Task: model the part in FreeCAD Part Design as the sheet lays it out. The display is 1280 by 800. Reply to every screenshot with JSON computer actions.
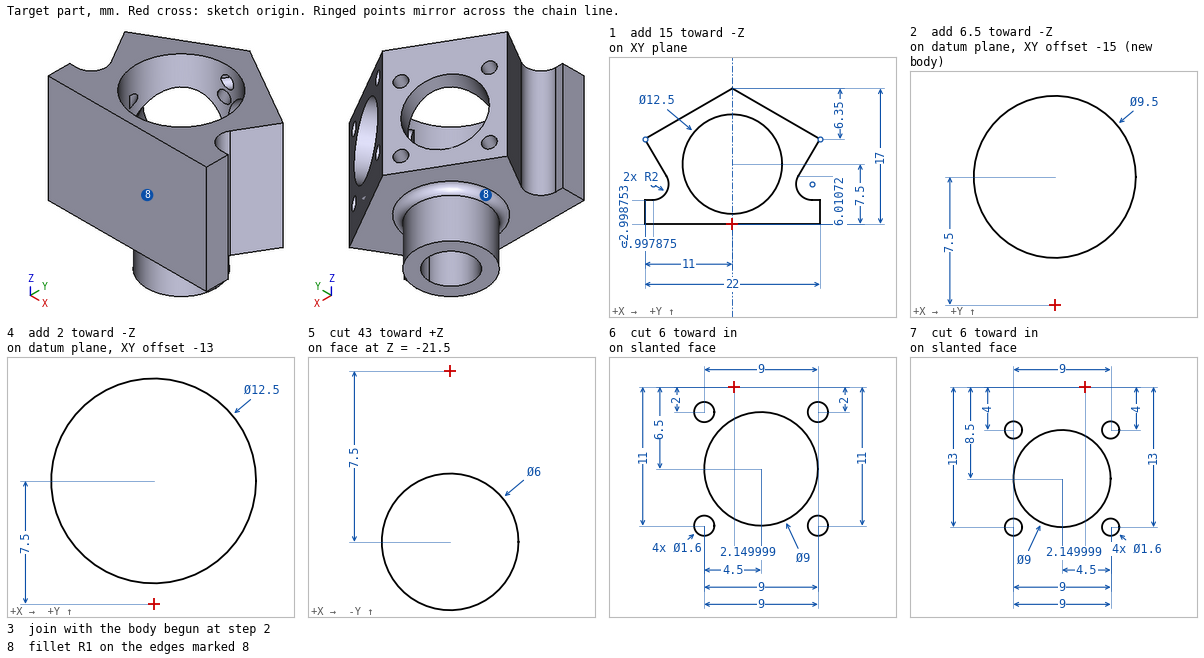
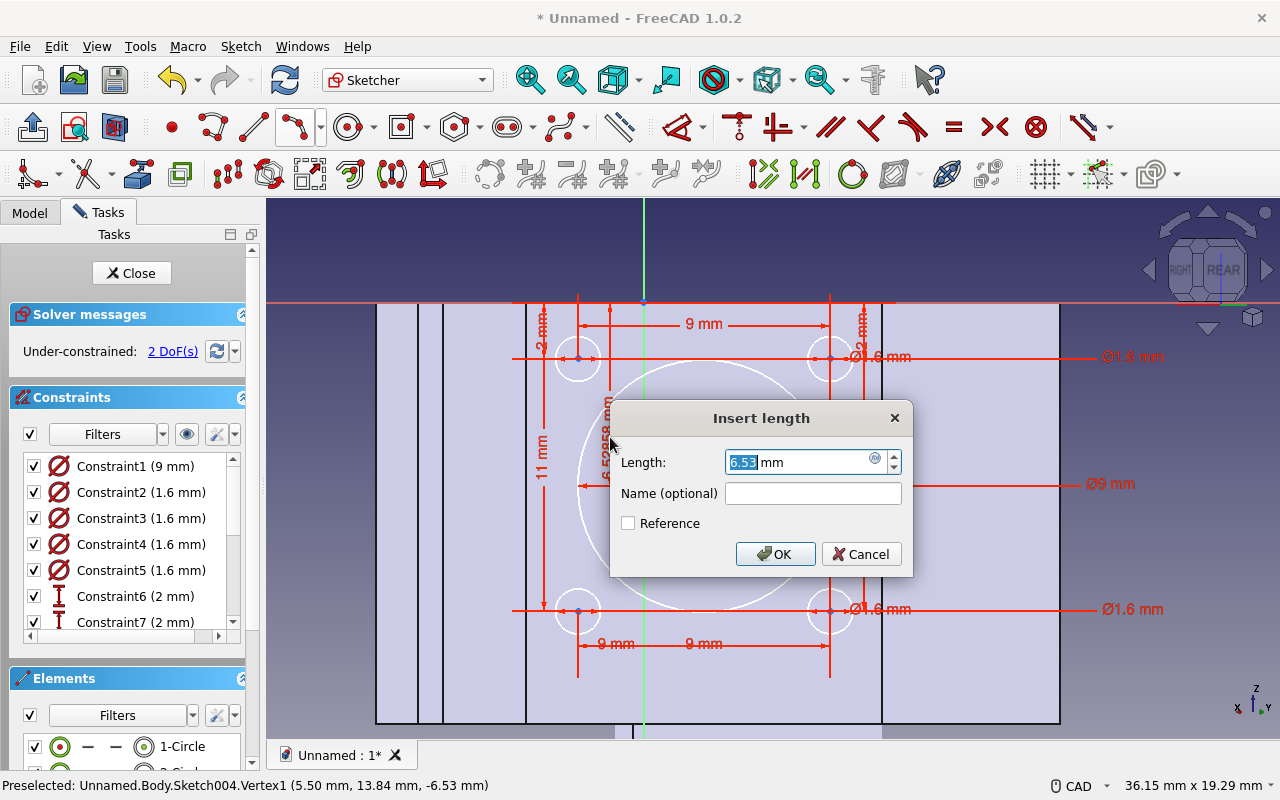
{"action": "type", "text": "6.5"}
{"action": "key", "text": "Return"}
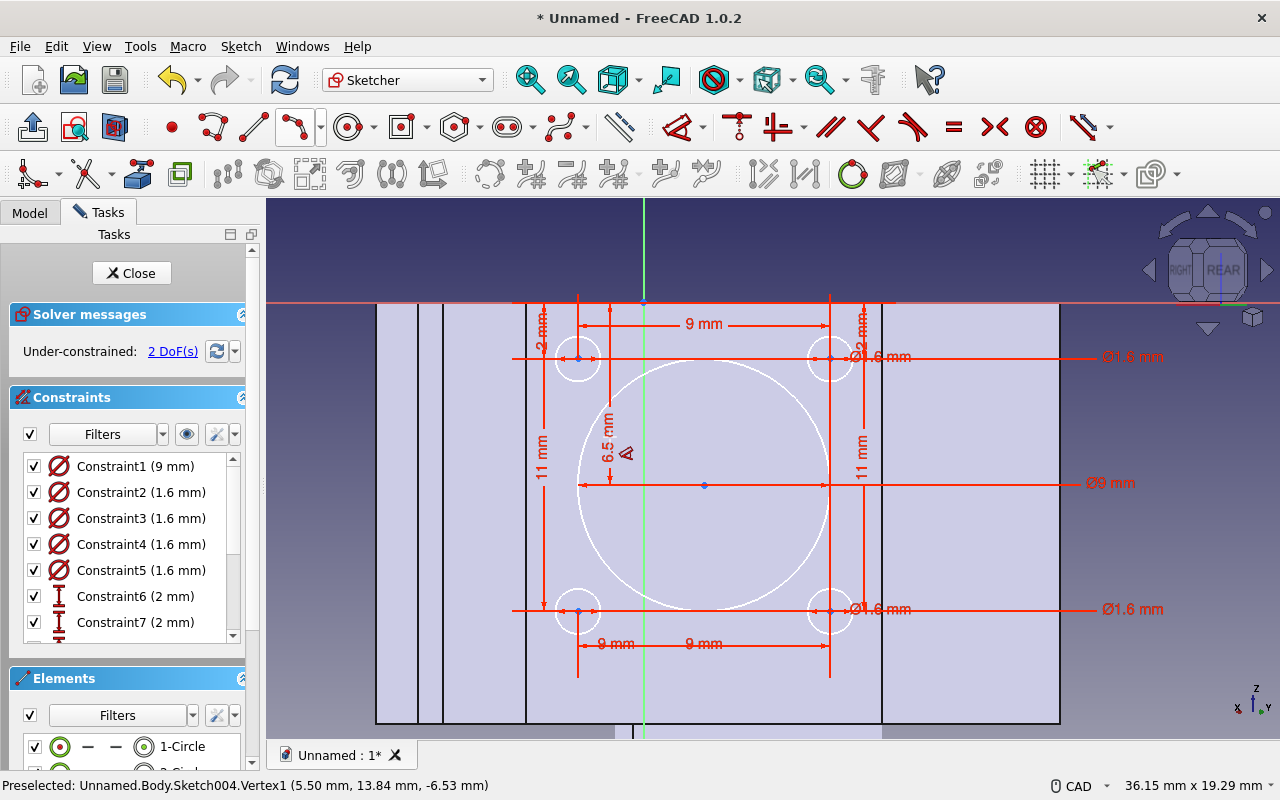
{"action": "left_click", "coordinate": [704, 485]}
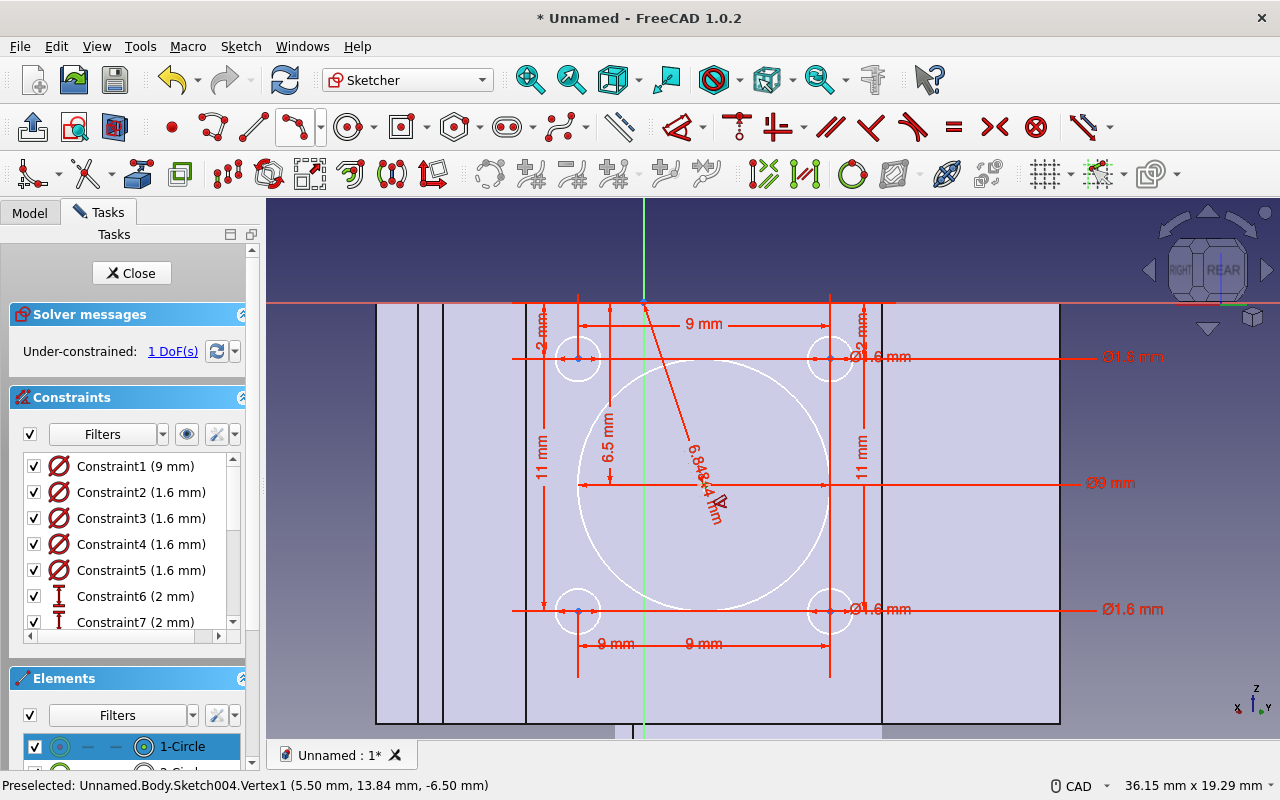
{"action": "left_click", "coordinate": [578, 611]}
{"action": "left_click", "coordinate": [685, 451]}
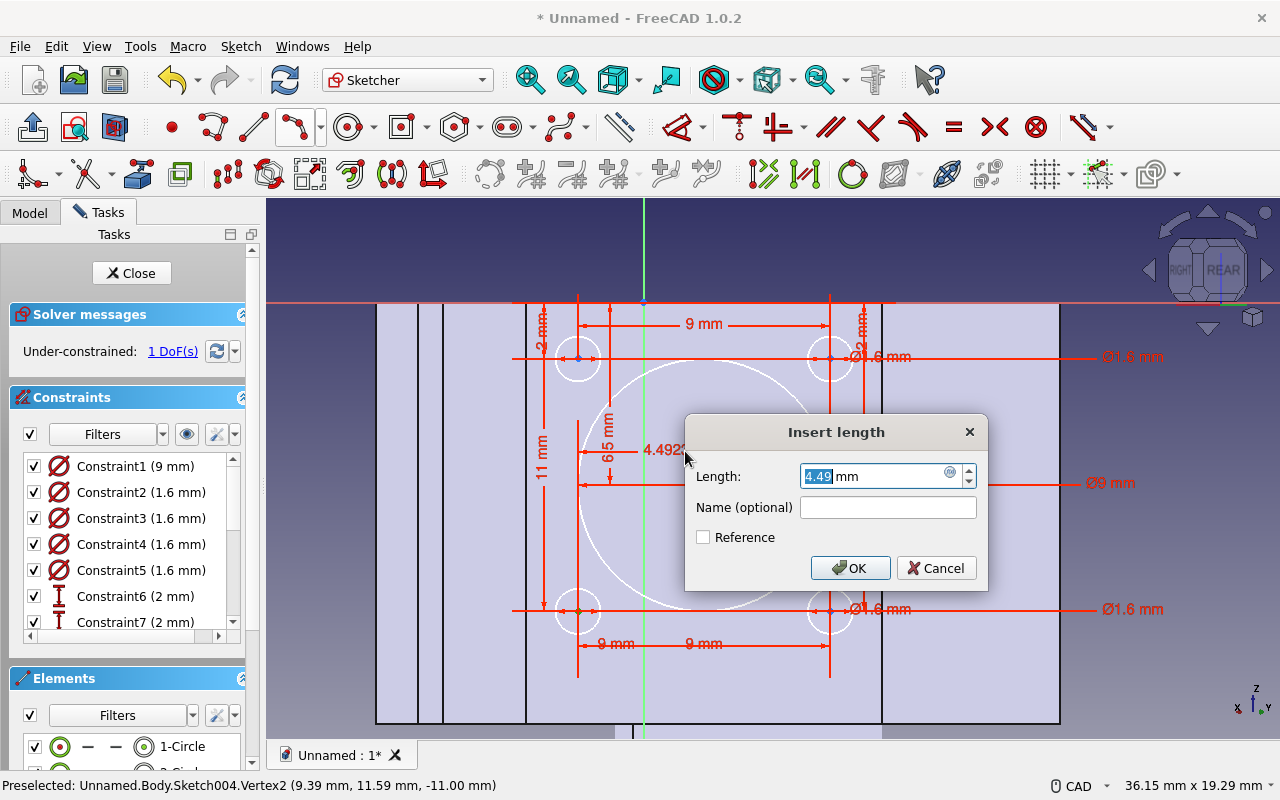
{"action": "type", "text": "4.5"}
{"action": "key", "text": "Return"}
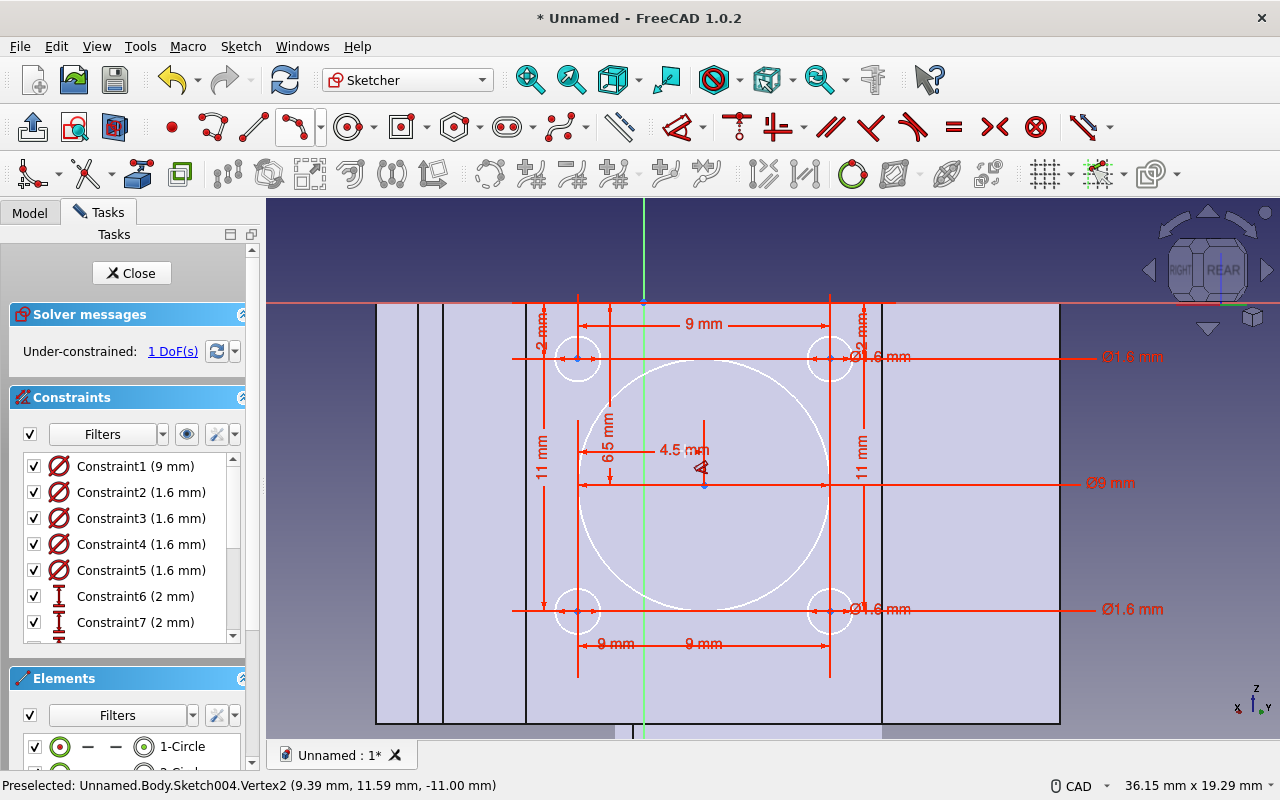
{"action": "left_click", "coordinate": [704, 485]}
{"action": "left_click", "coordinate": [674, 269]}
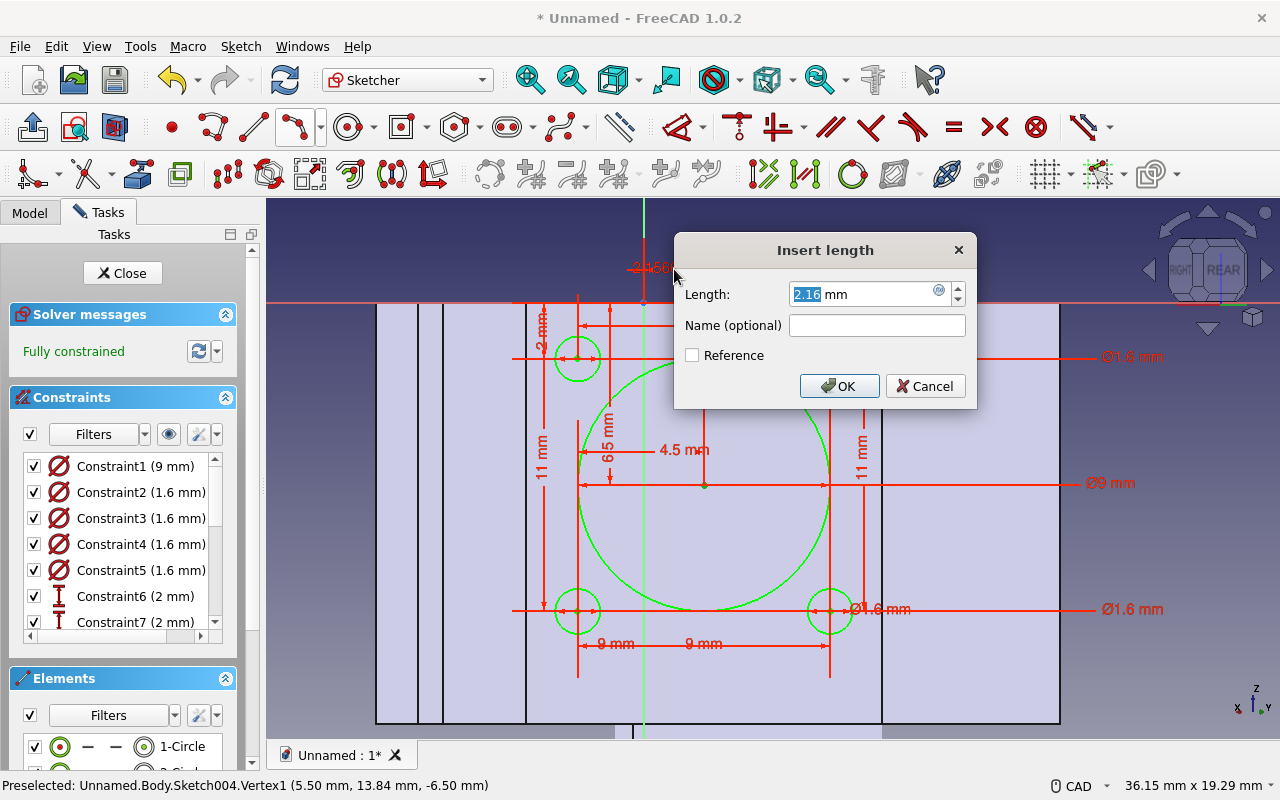
{"action": "type", "text": "2.149999"}
{"action": "key", "text": "Return"}
{"action": "key", "text": "Escape"}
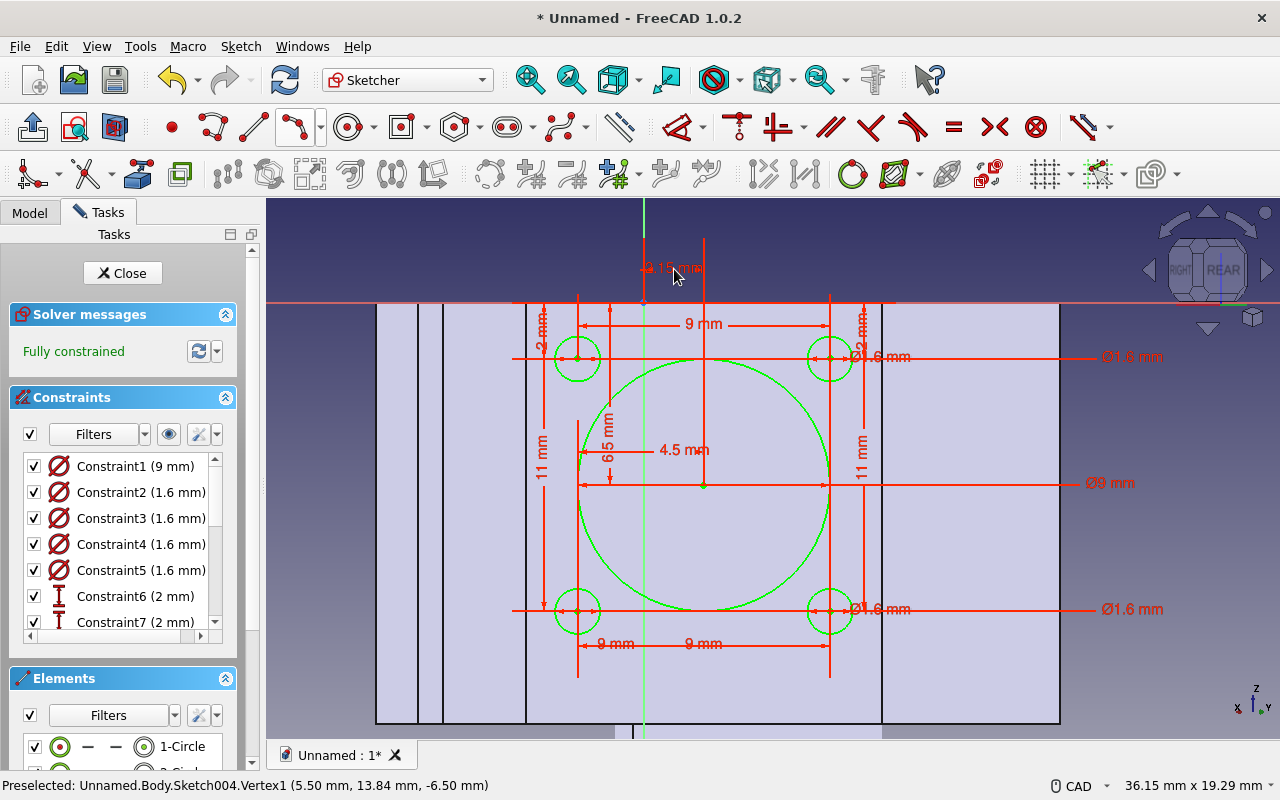
{"action": "left_click", "coordinate": [123, 273]}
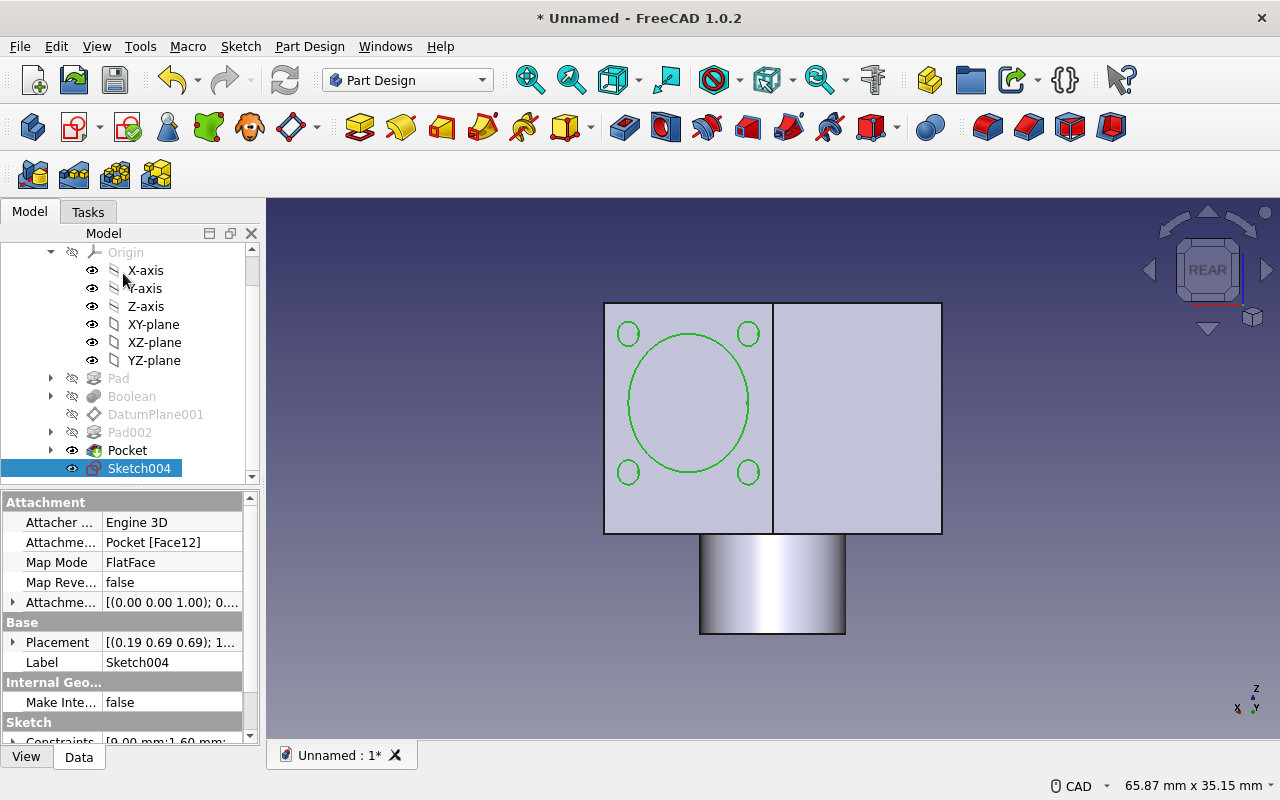
{"action": "left_click", "coordinate": [625, 128]}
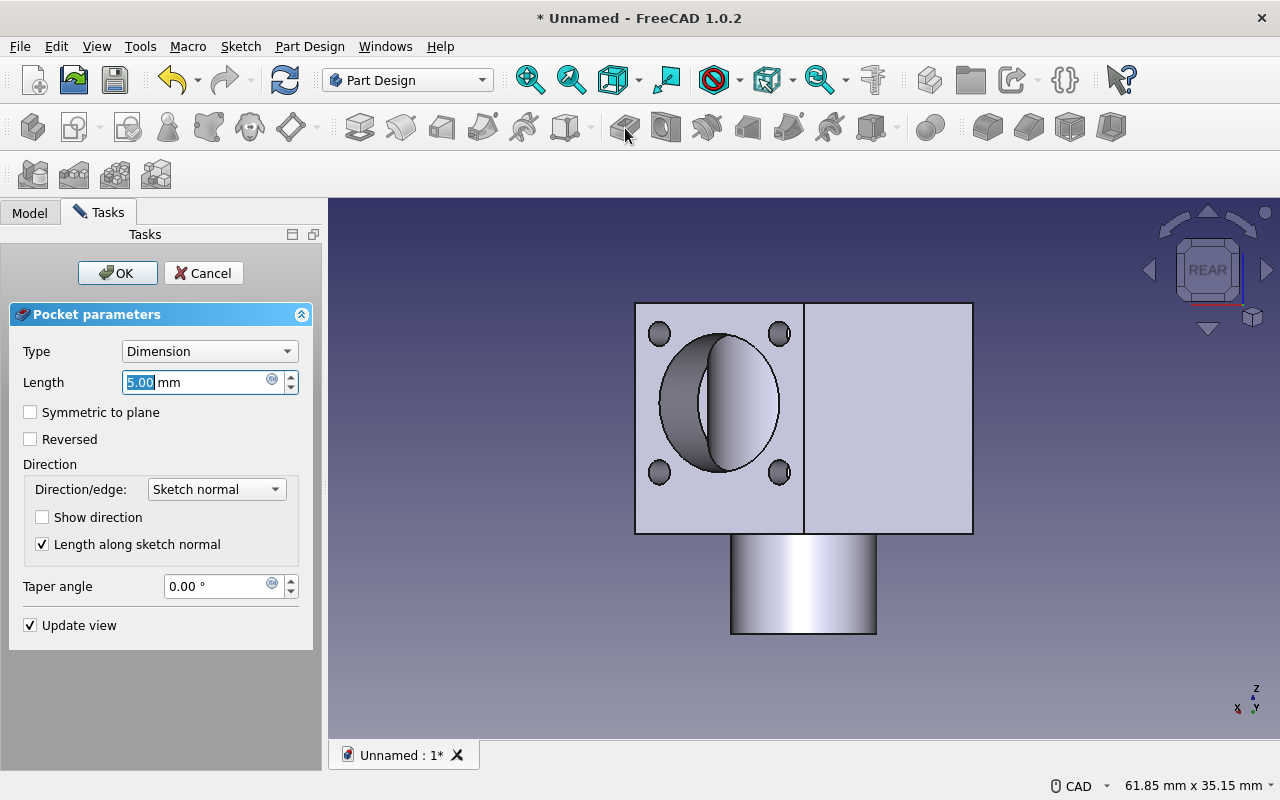
{"action": "type", "text": "6"}
{"action": "key", "text": "Tab"}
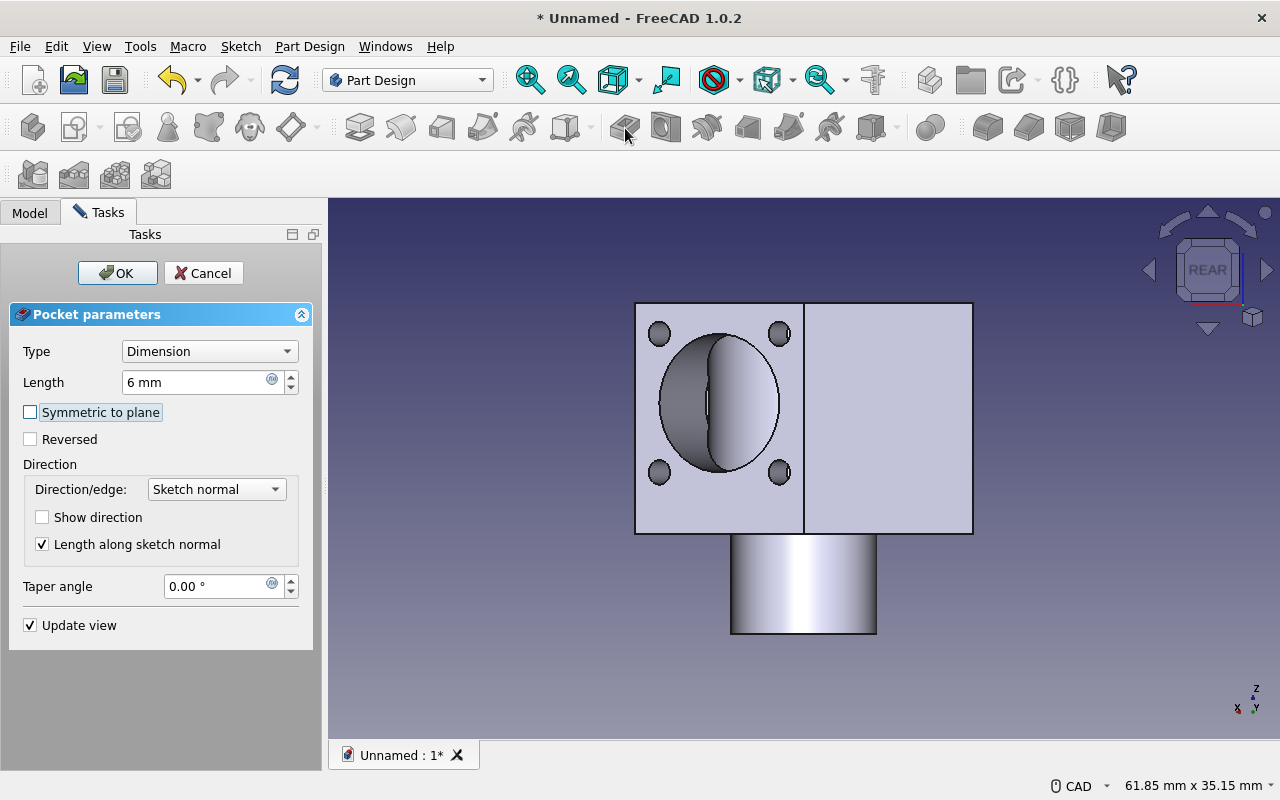
{"action": "left_click", "coordinate": [118, 273]}